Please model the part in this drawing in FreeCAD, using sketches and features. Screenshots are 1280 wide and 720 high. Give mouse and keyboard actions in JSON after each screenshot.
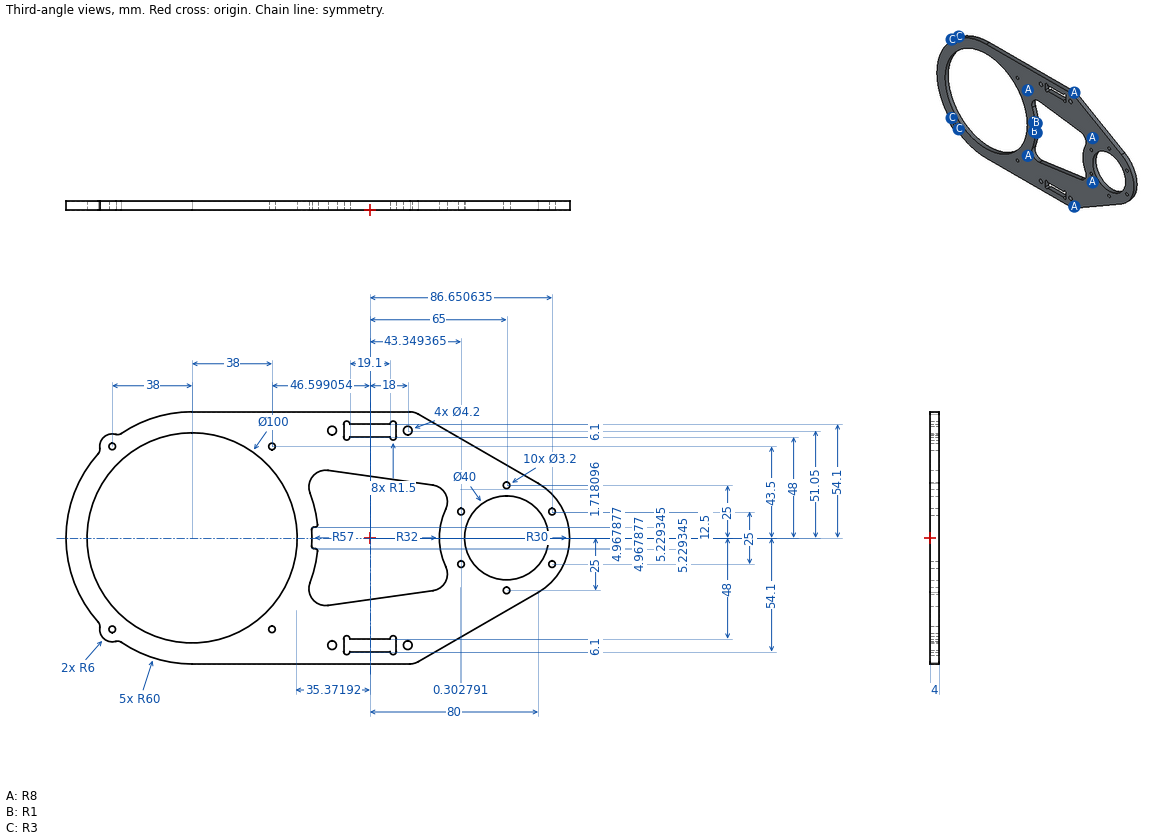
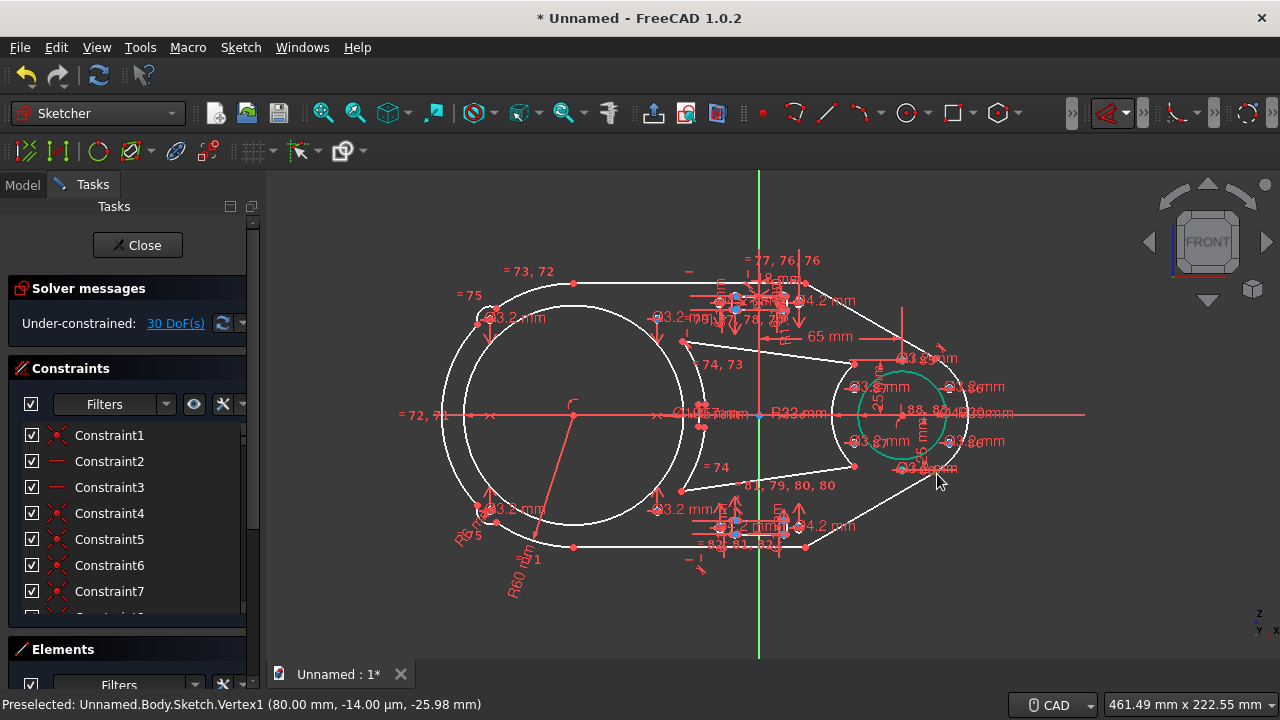
{"action": "key", "text": "l"}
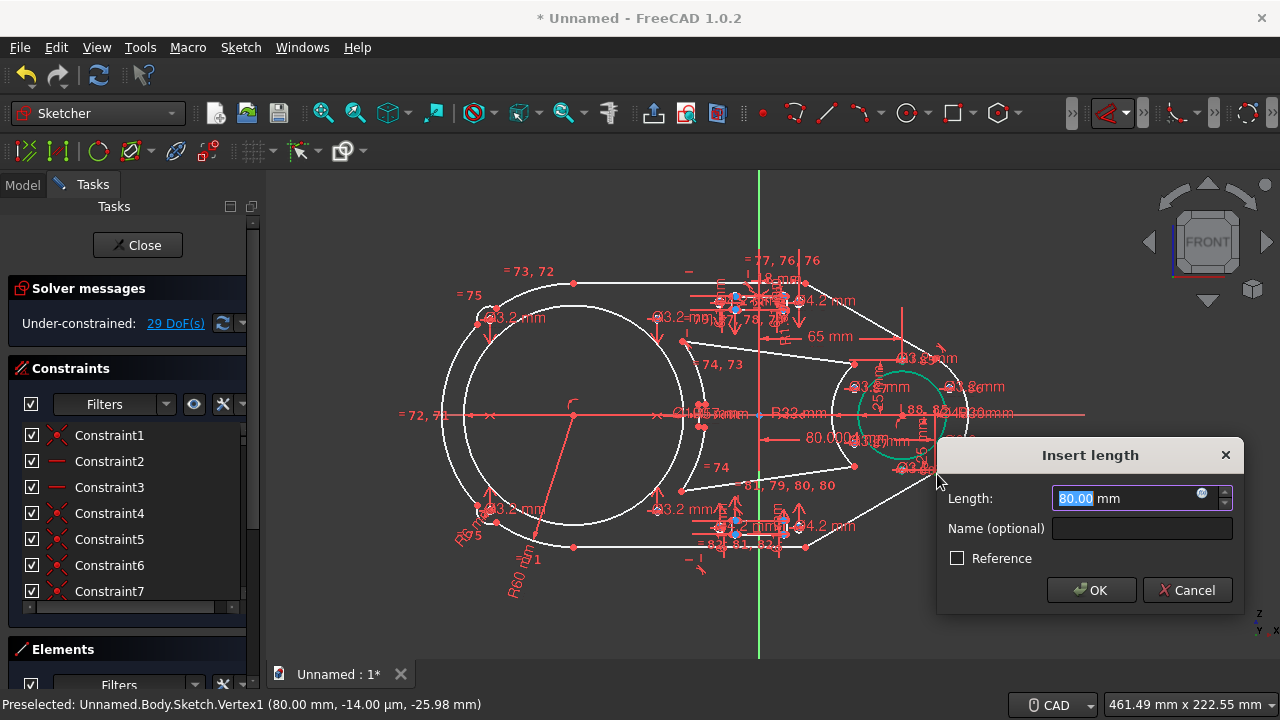
{"action": "type", "text": "80"}
{"action": "key", "text": "Return"}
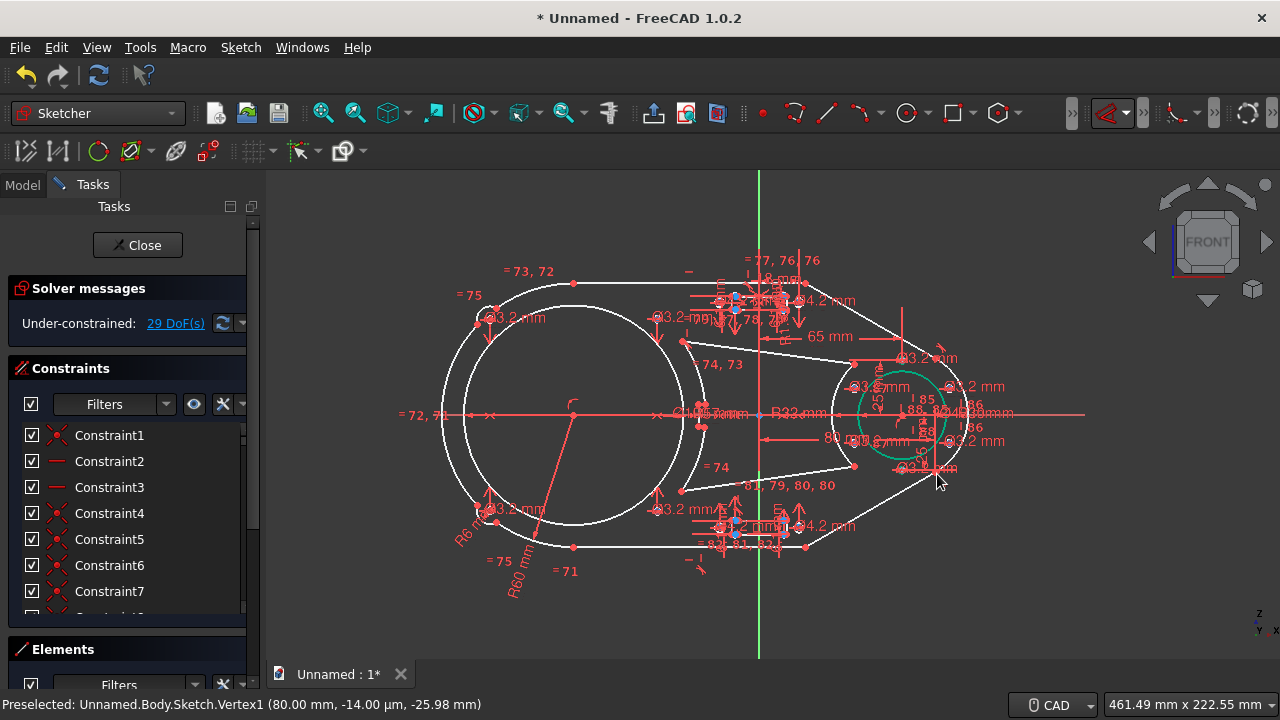
{"action": "left_click", "coordinate": [935, 358]}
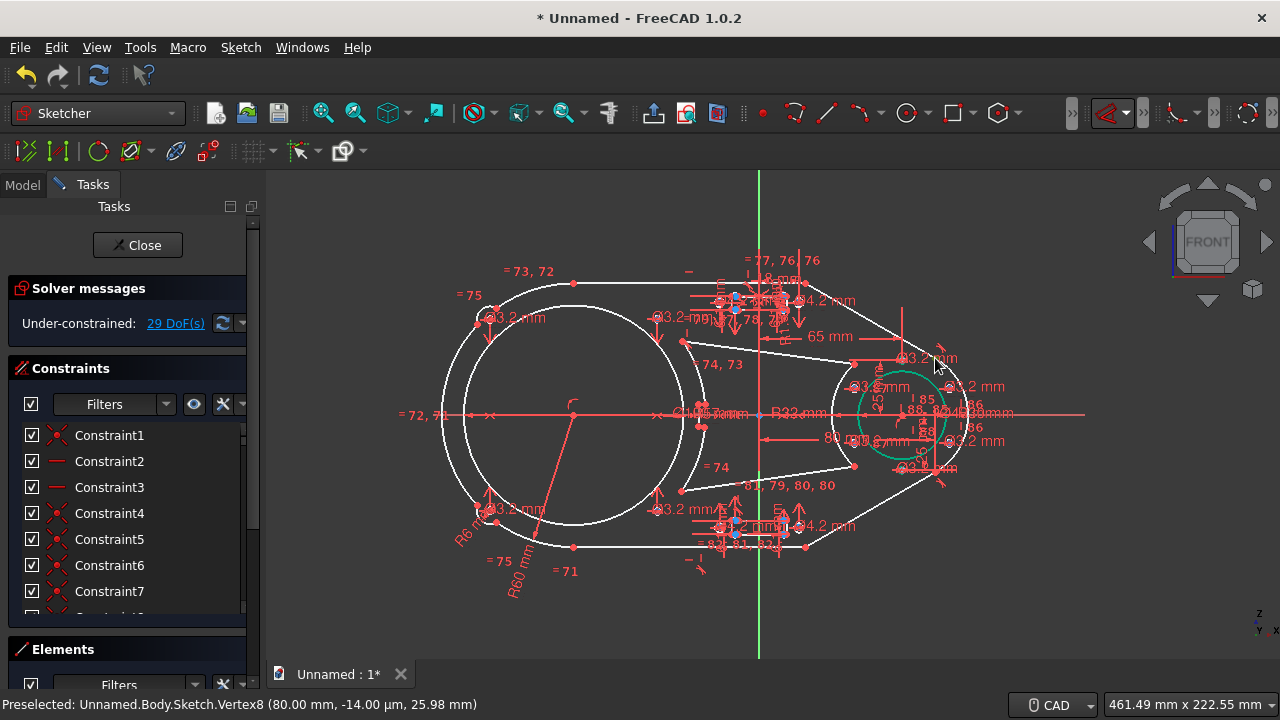
{"action": "left_click", "coordinate": [1128, 114]}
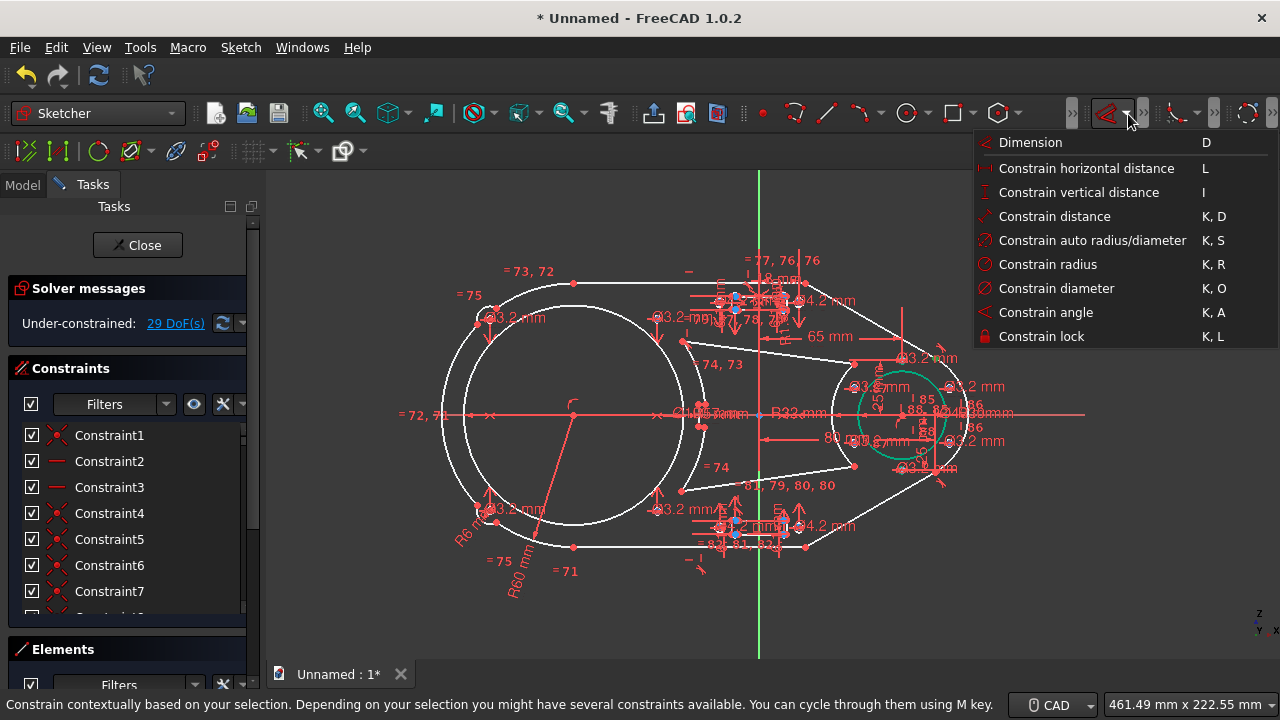
{"action": "left_click", "coordinate": [1126, 168]}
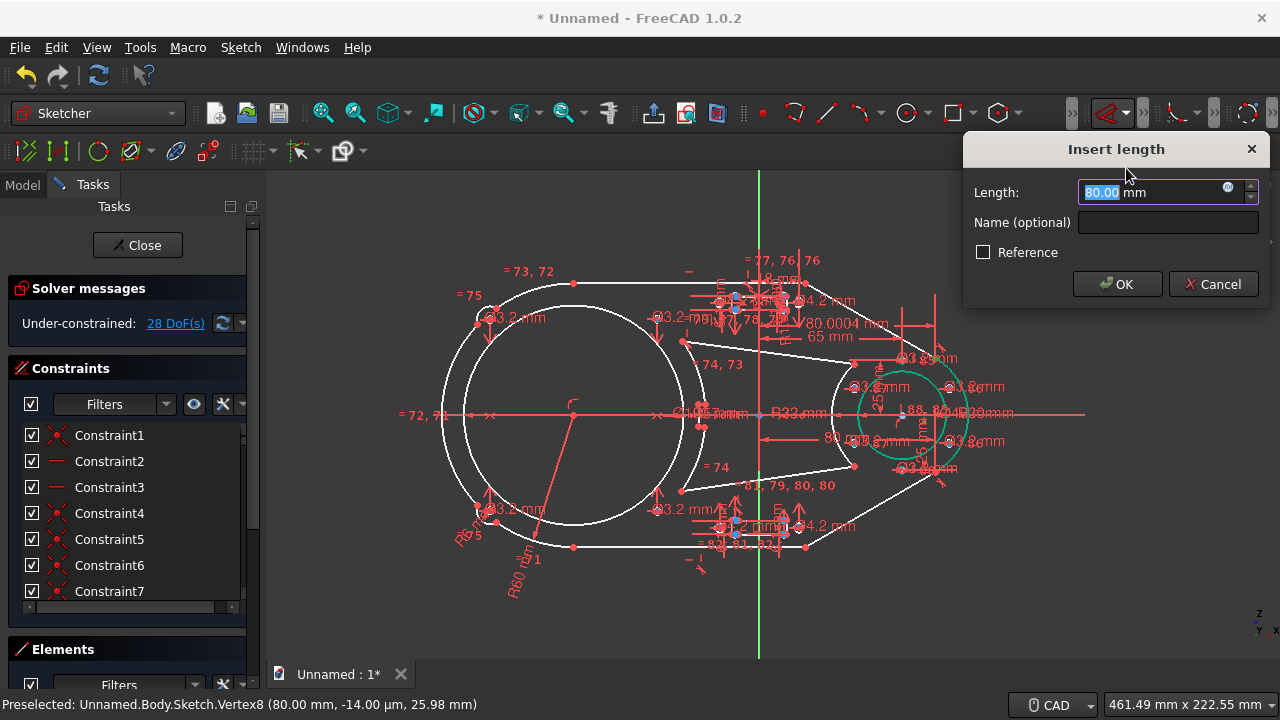
{"action": "type", "text": "80"}
{"action": "key", "text": "Return"}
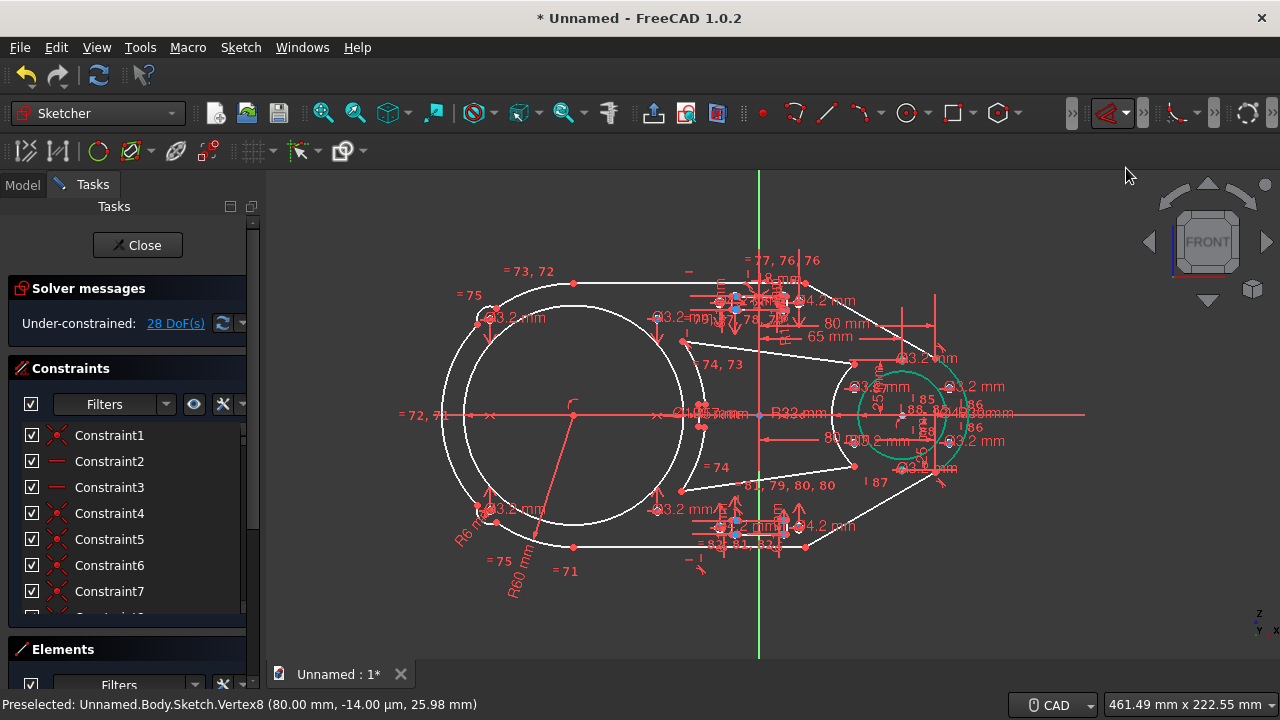
{"action": "scroll", "coordinate": [738, 310], "scroll_direction": "up", "scroll_amount": 7}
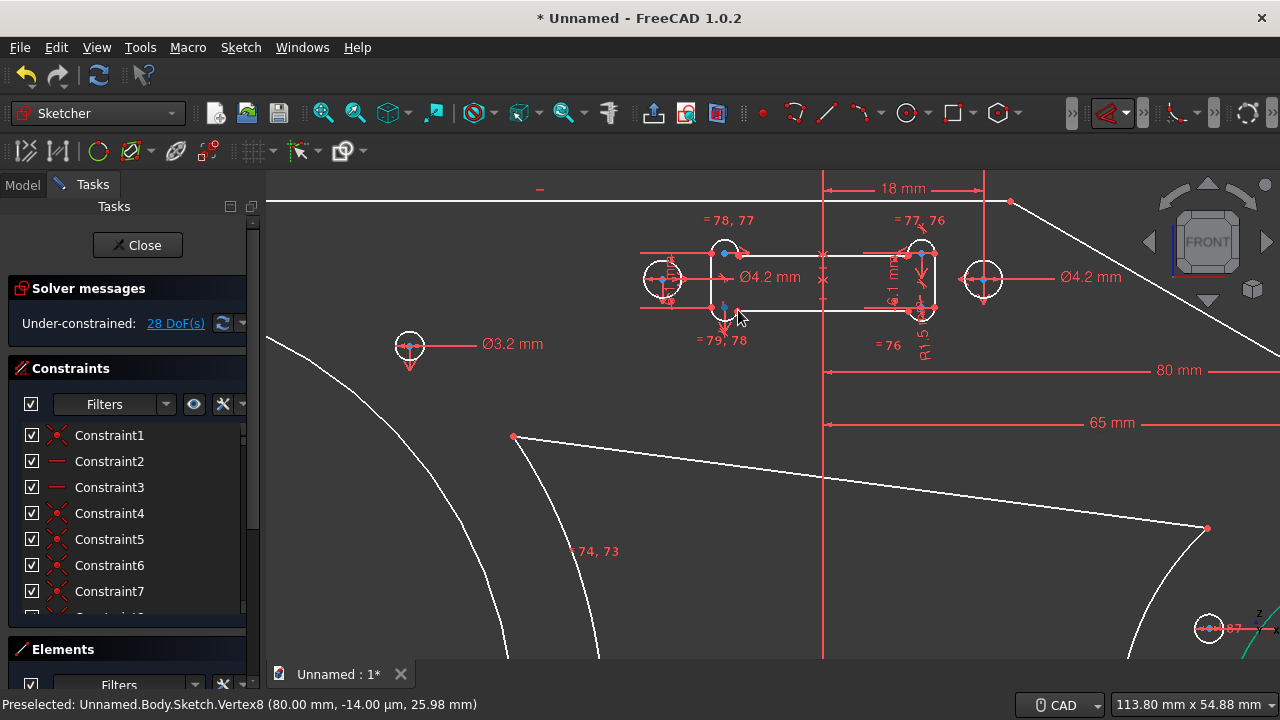
{"action": "left_click", "coordinate": [738, 311]}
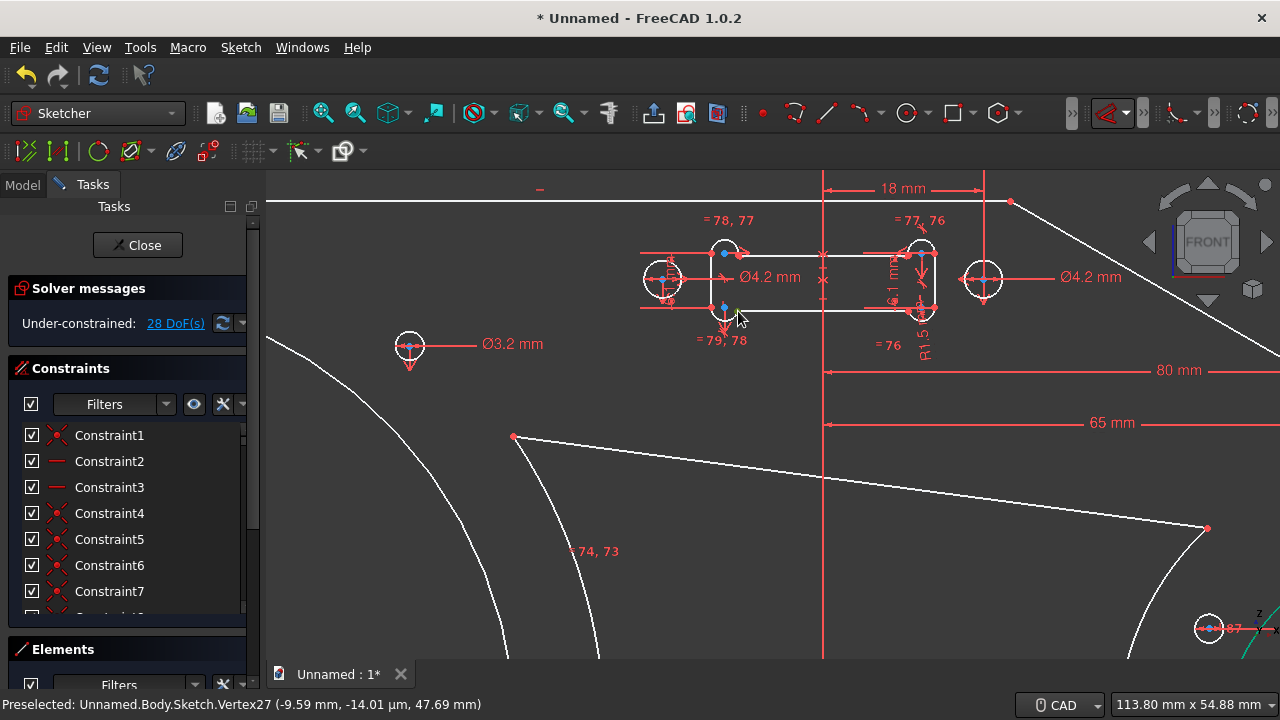
{"action": "key", "text": "i"}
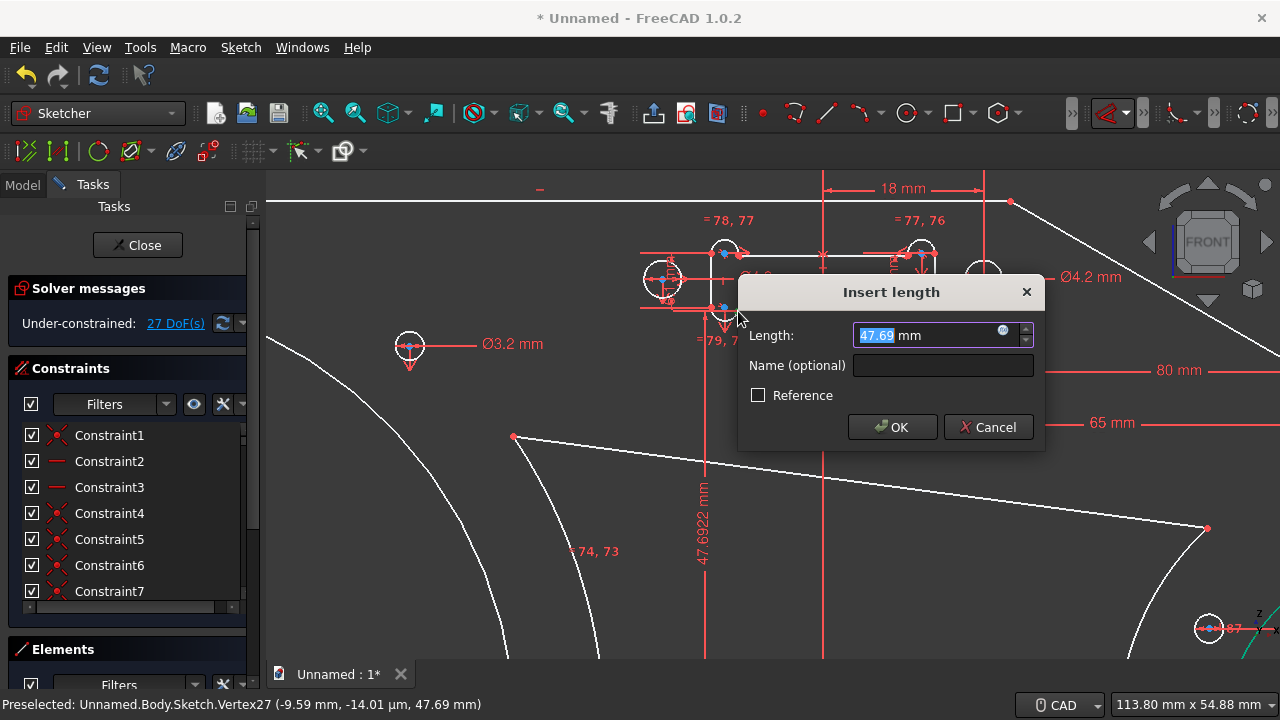
{"action": "type", "text": "48"}
{"action": "key", "text": "Return"}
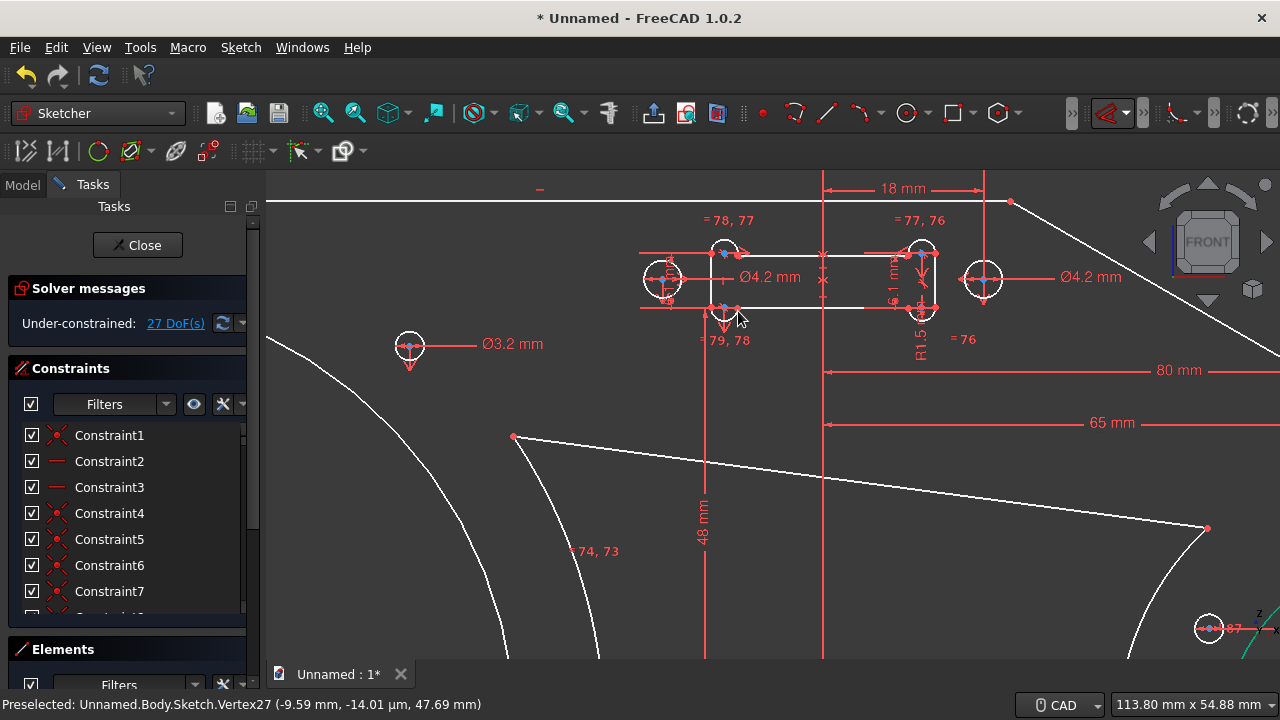
{"action": "left_click", "coordinate": [935, 308]}